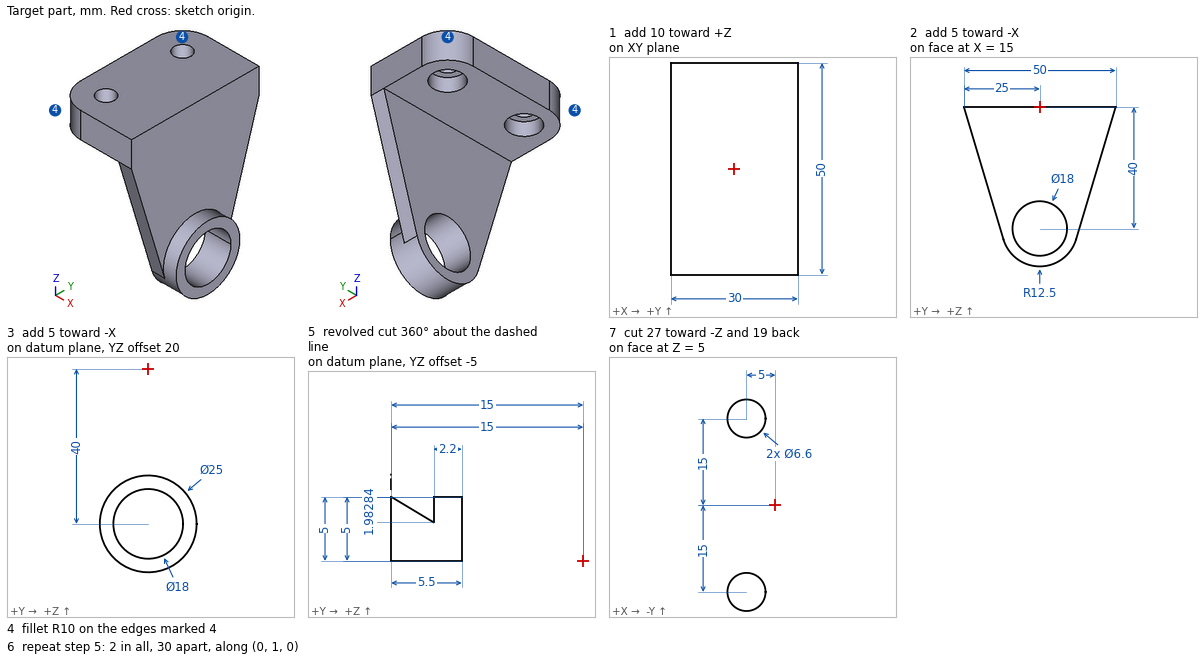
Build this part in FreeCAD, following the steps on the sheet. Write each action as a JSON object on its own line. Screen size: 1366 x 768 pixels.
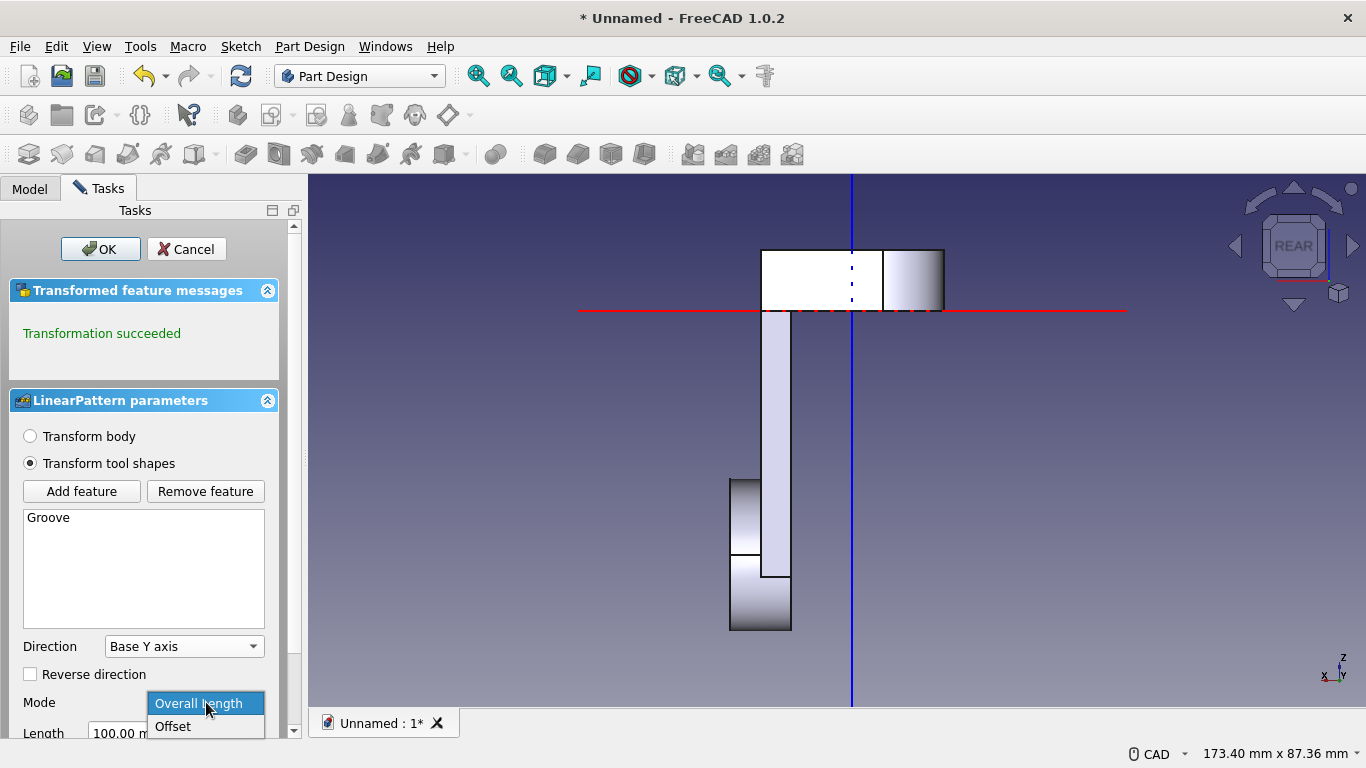
{"action": "left_click", "coordinate": [204, 726]}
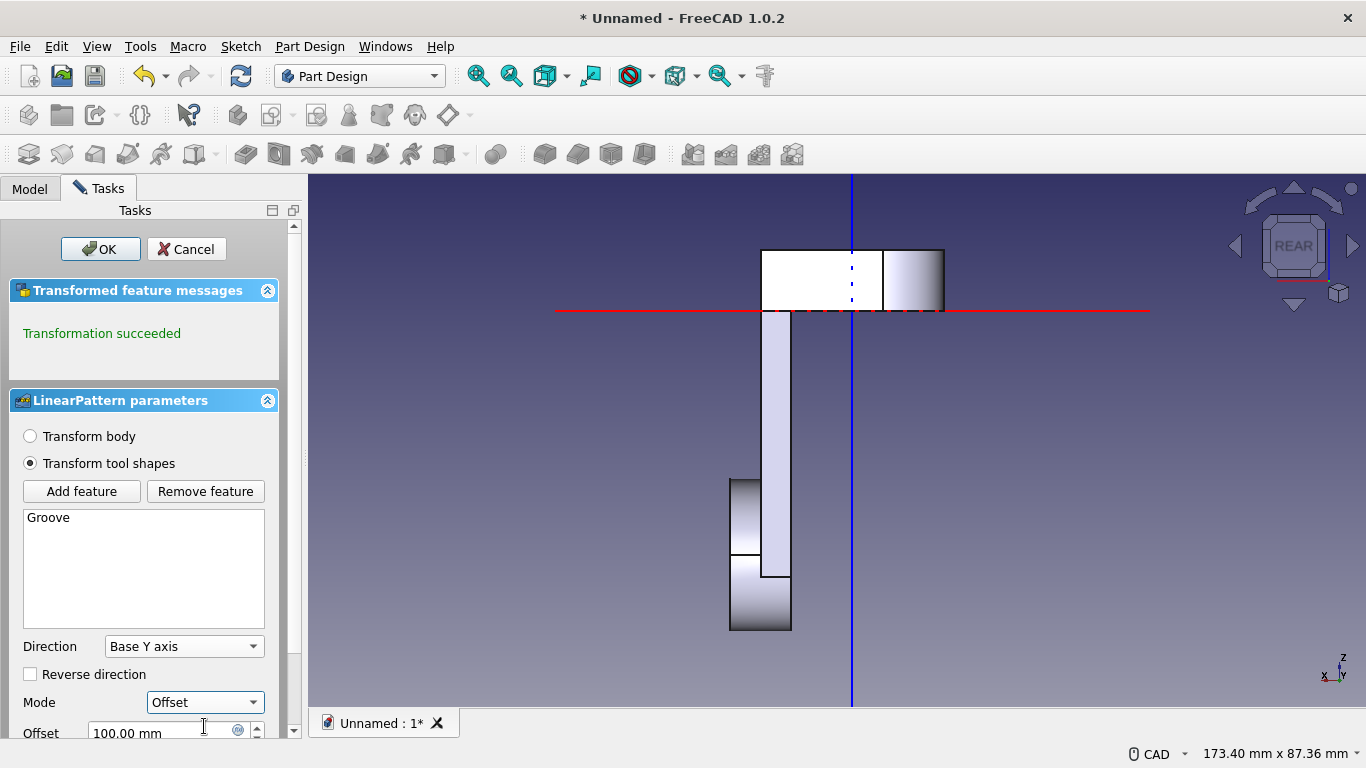
{"action": "scroll", "coordinate": [294, 479], "scroll_direction": "down", "scroll_amount": 2}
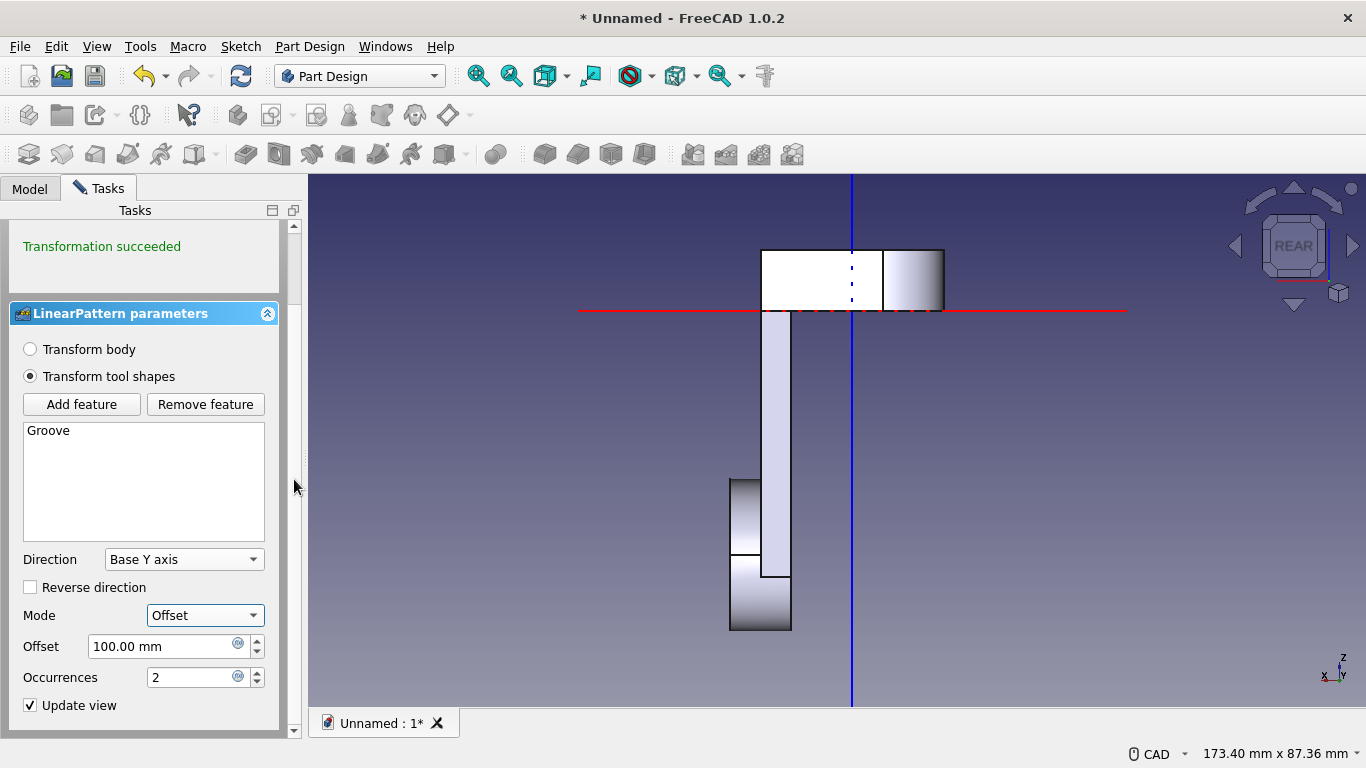
{"action": "triple_click", "coordinate": [170, 646]}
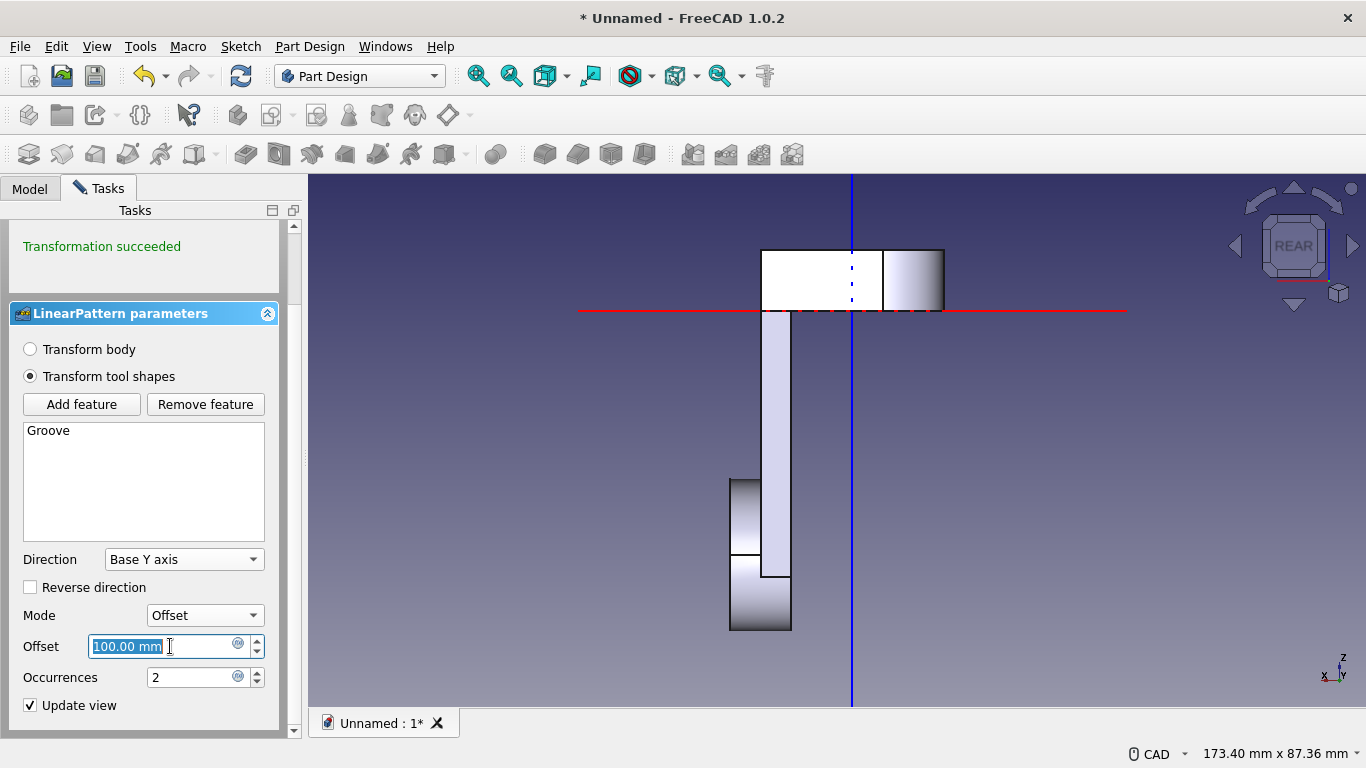
{"action": "type", "text": "30"}
{"action": "key", "text": "Tab"}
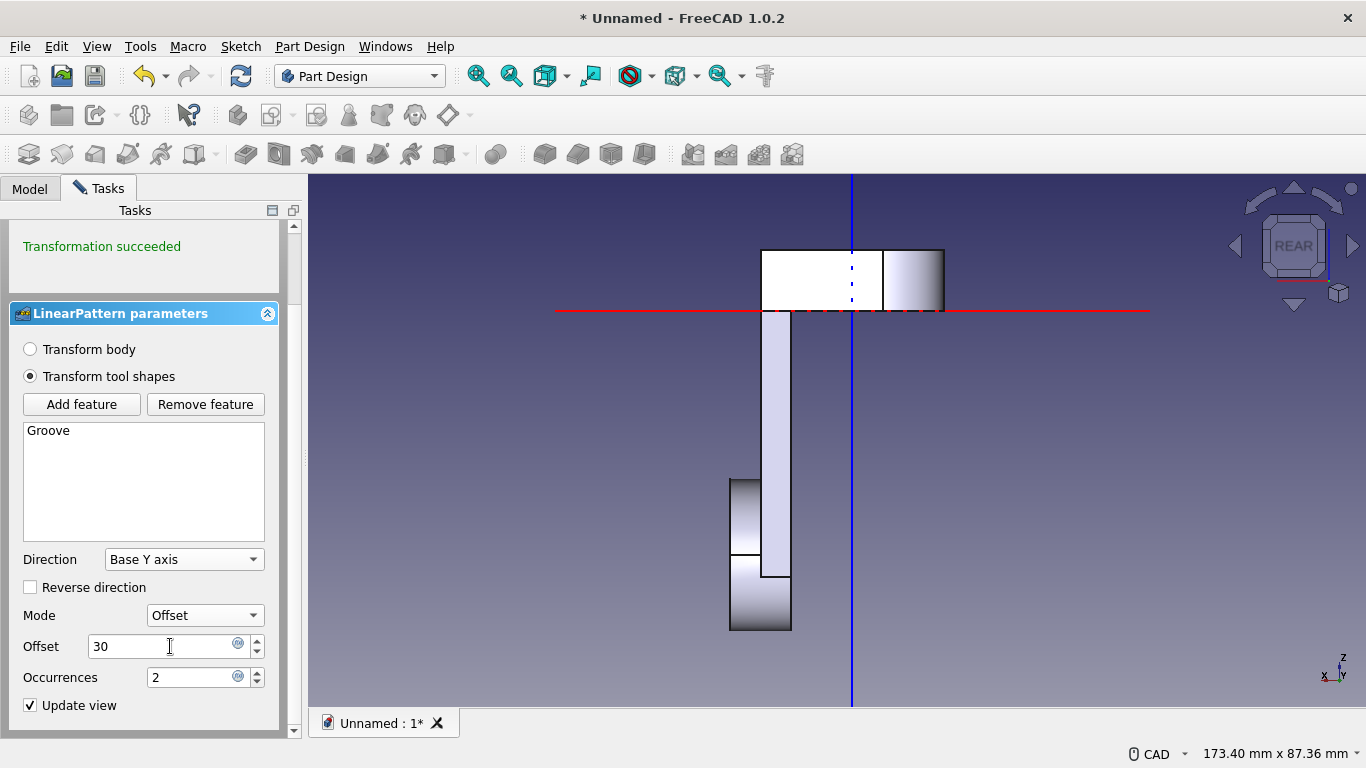
{"action": "triple_click", "coordinate": [199, 678]}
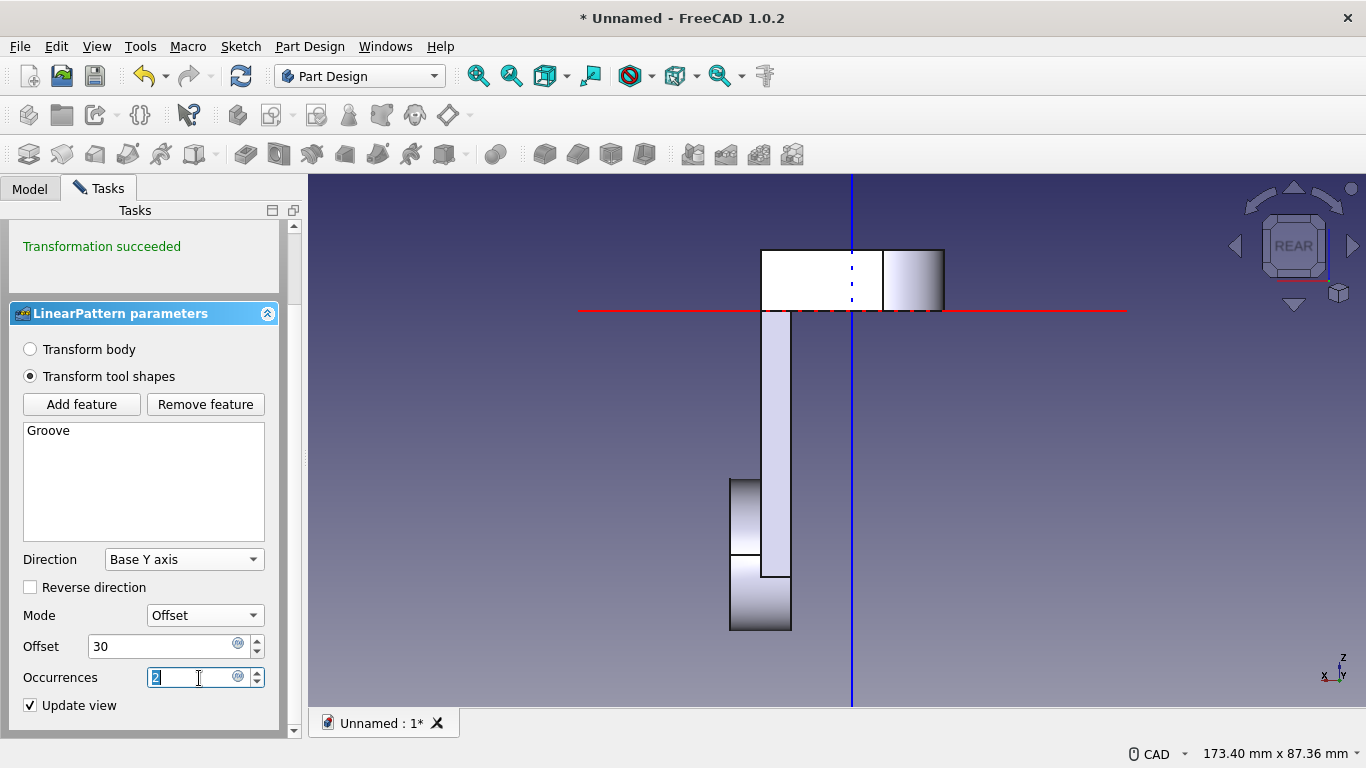
{"action": "type", "text": "2"}
{"action": "key", "text": "Tab"}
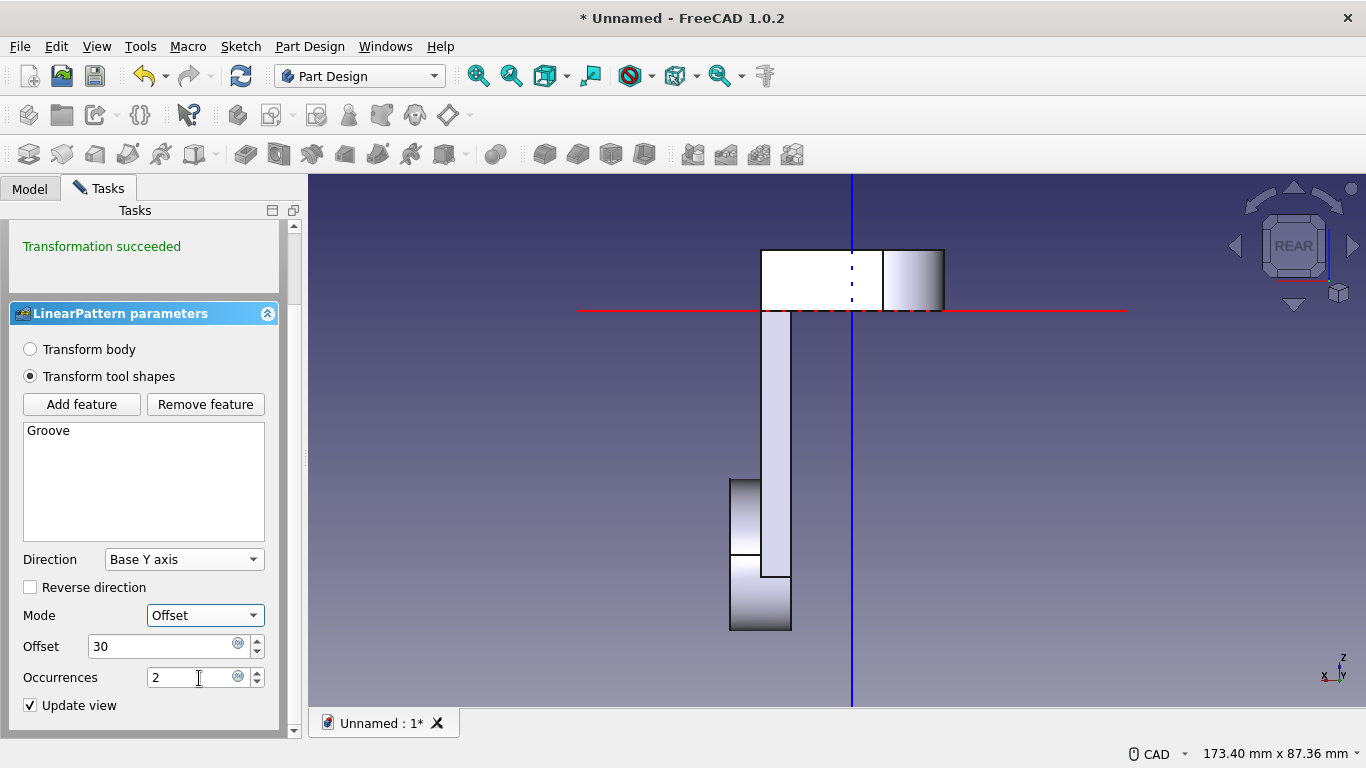
{"action": "scroll", "coordinate": [294, 479], "scroll_direction": "up", "scroll_amount": 3}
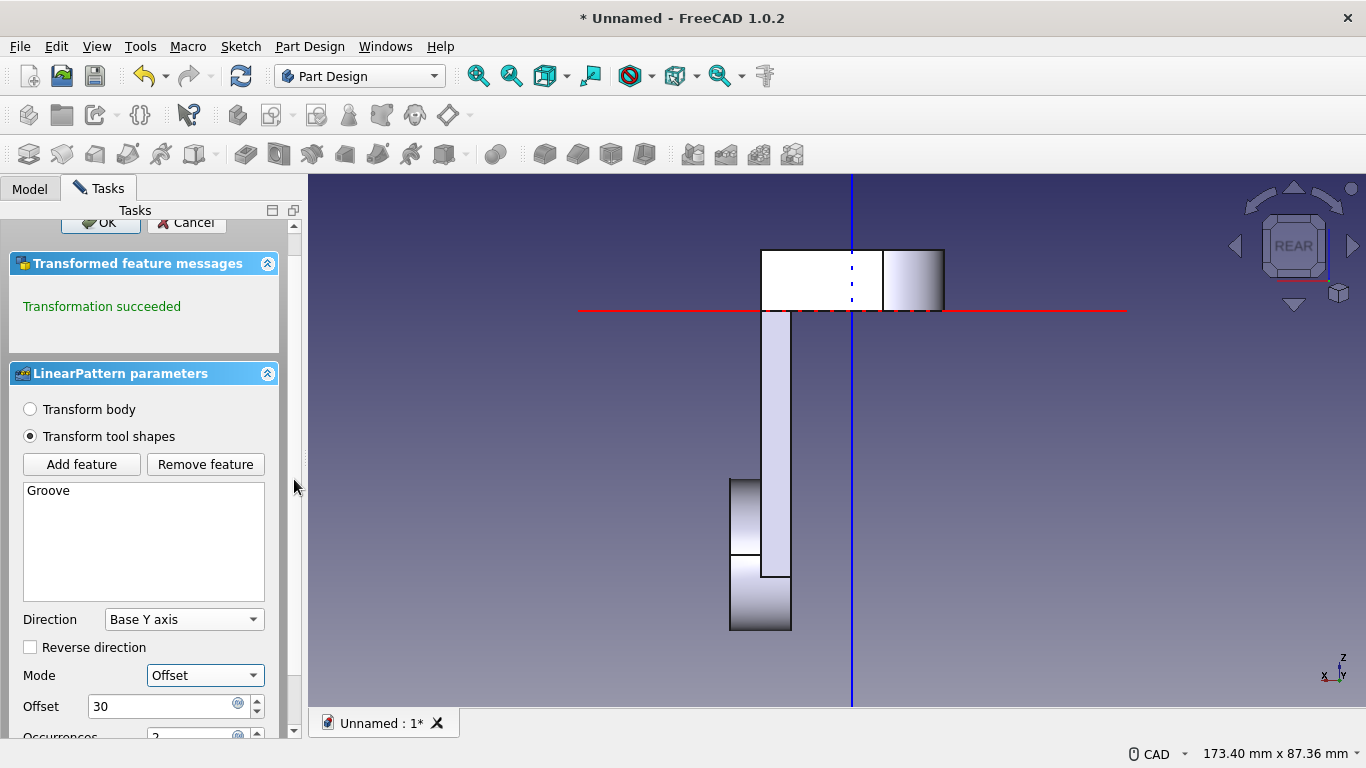
{"action": "left_click", "coordinate": [101, 249]}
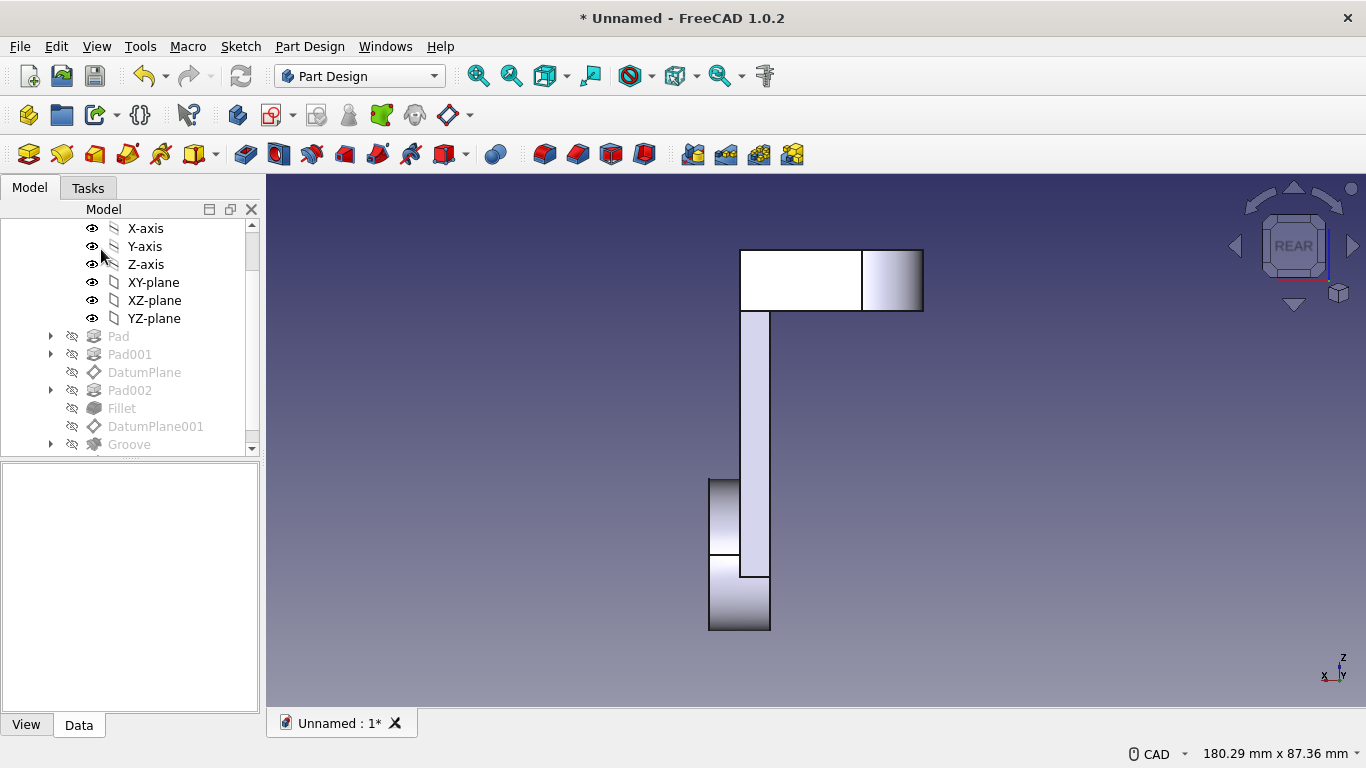
{"action": "key", "text": "5"}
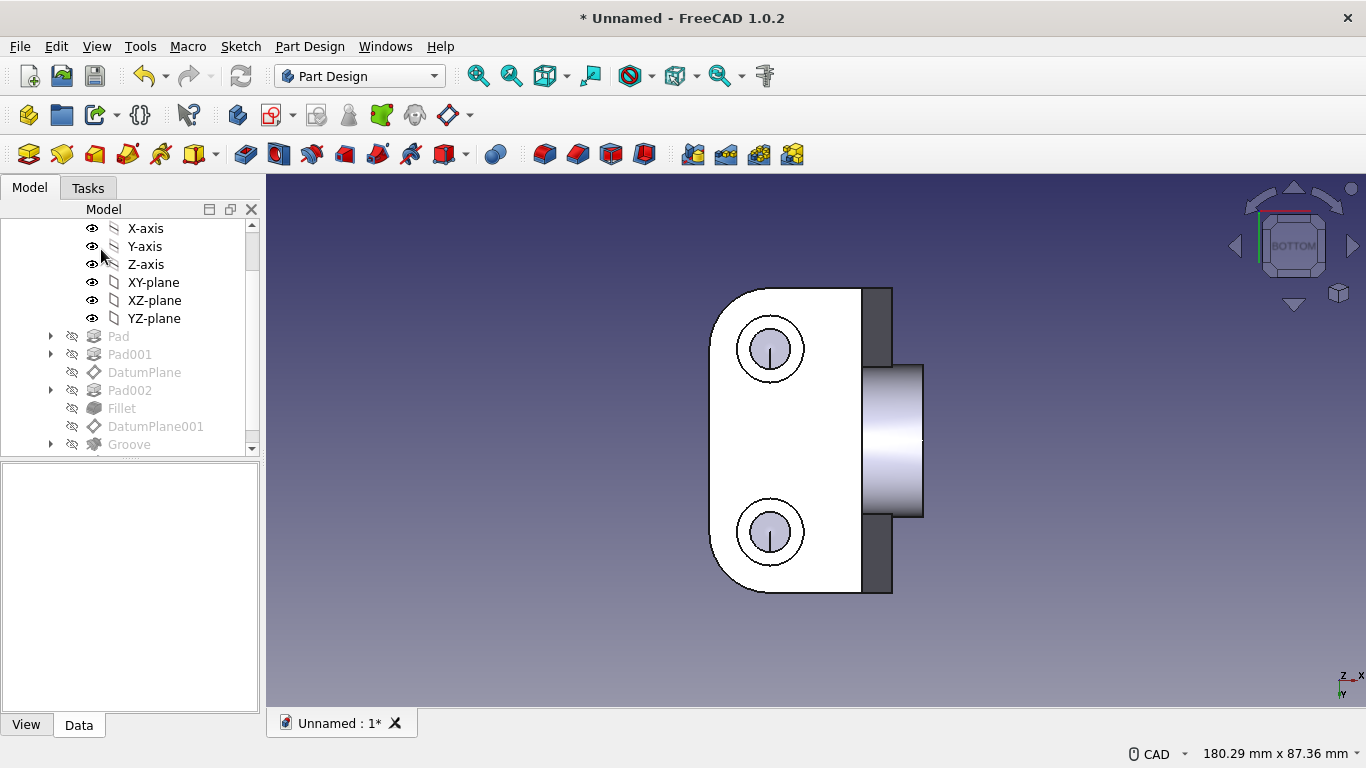
{"action": "scroll", "coordinate": [789, 512], "scroll_direction": "up", "scroll_amount": 4}